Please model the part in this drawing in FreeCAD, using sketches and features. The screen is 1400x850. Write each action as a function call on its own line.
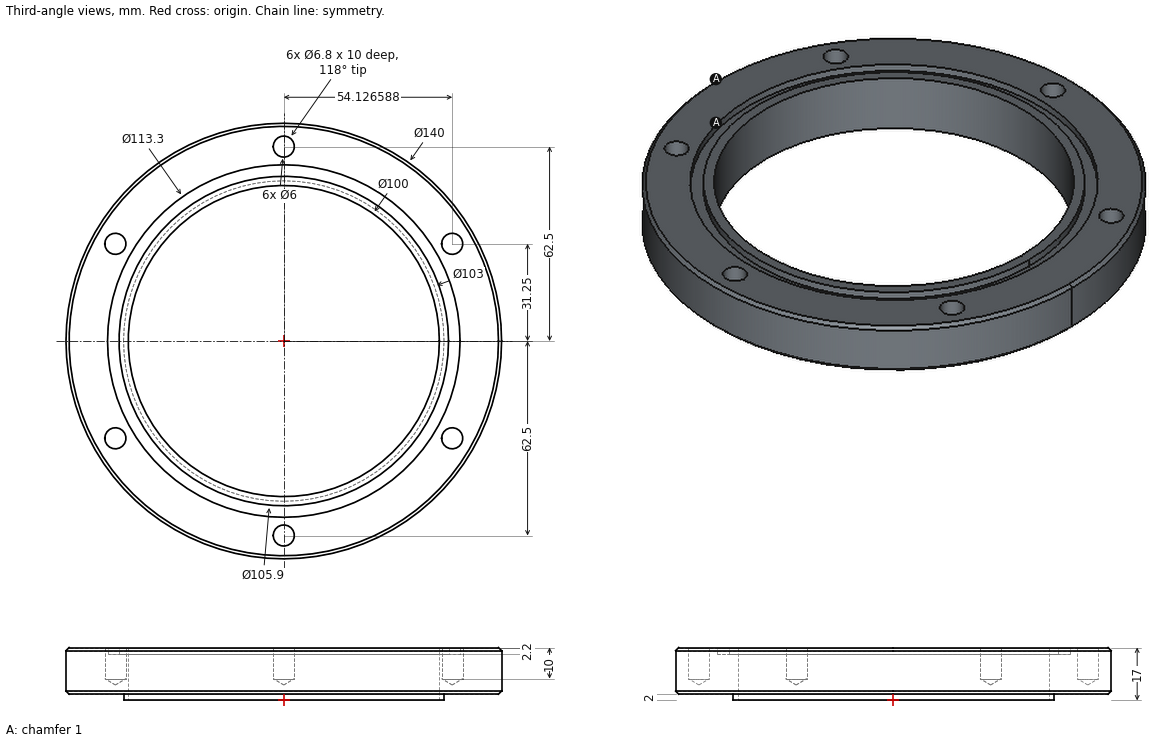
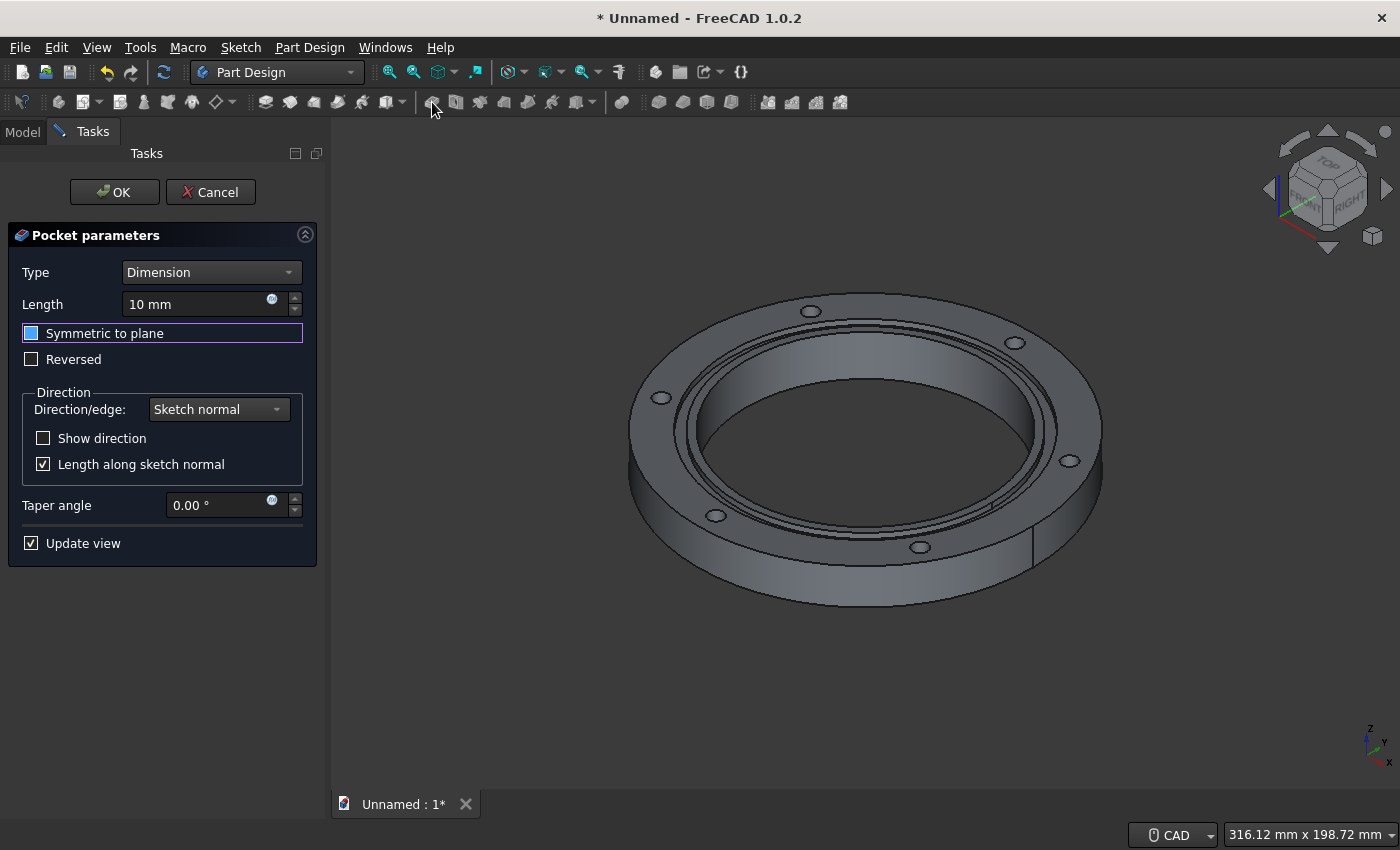
click(115, 192)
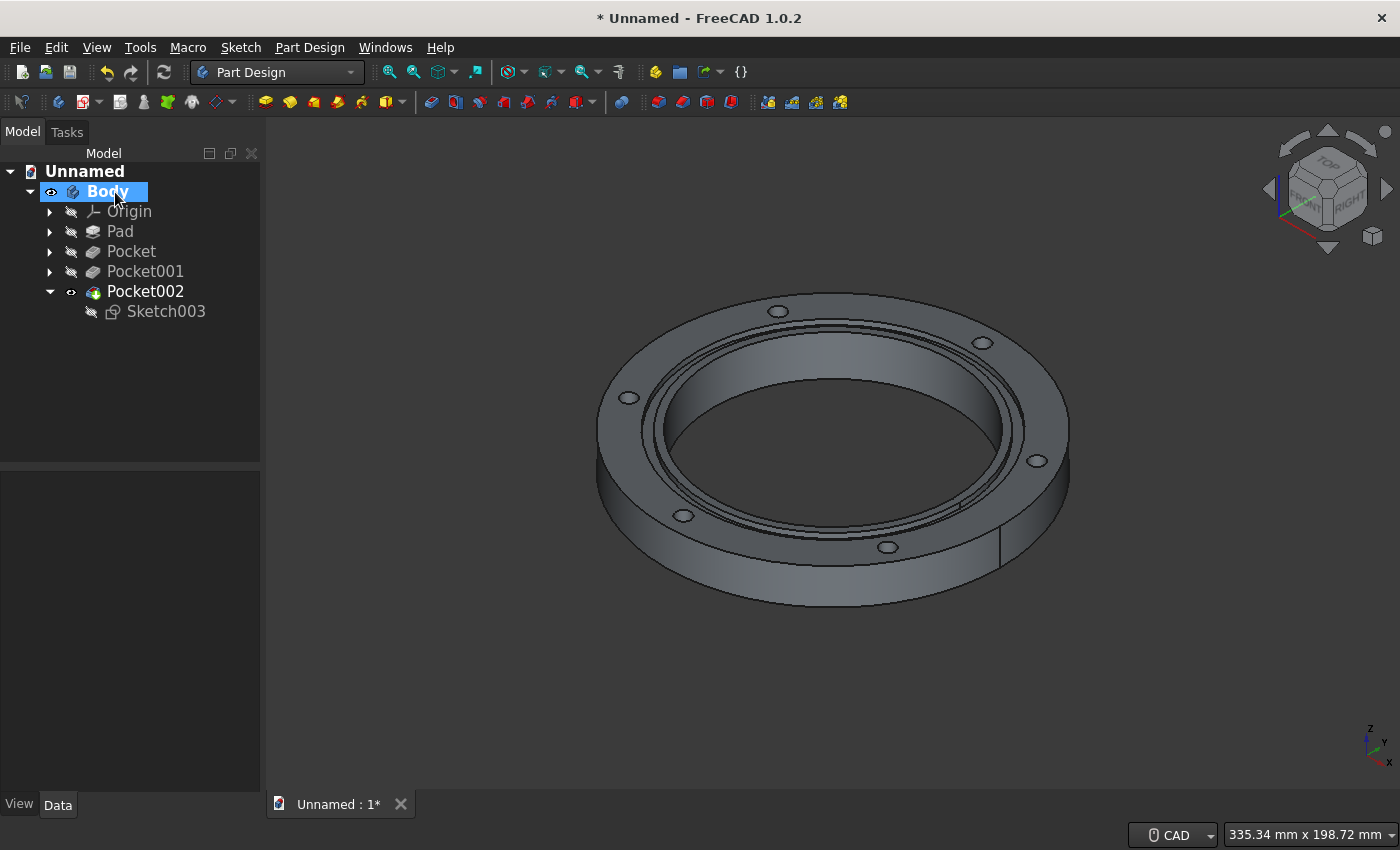
click(1024, 373)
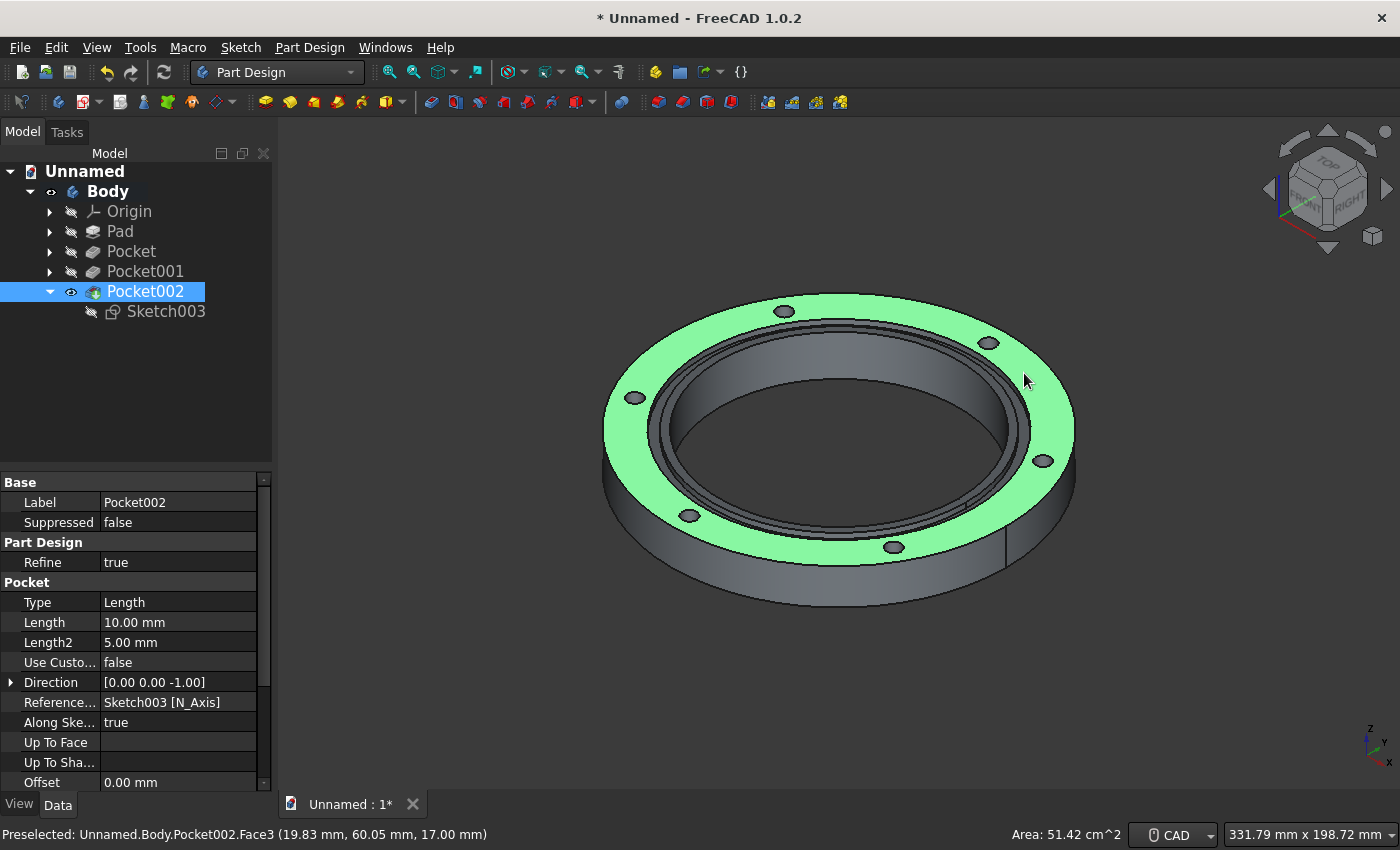
click(84, 102)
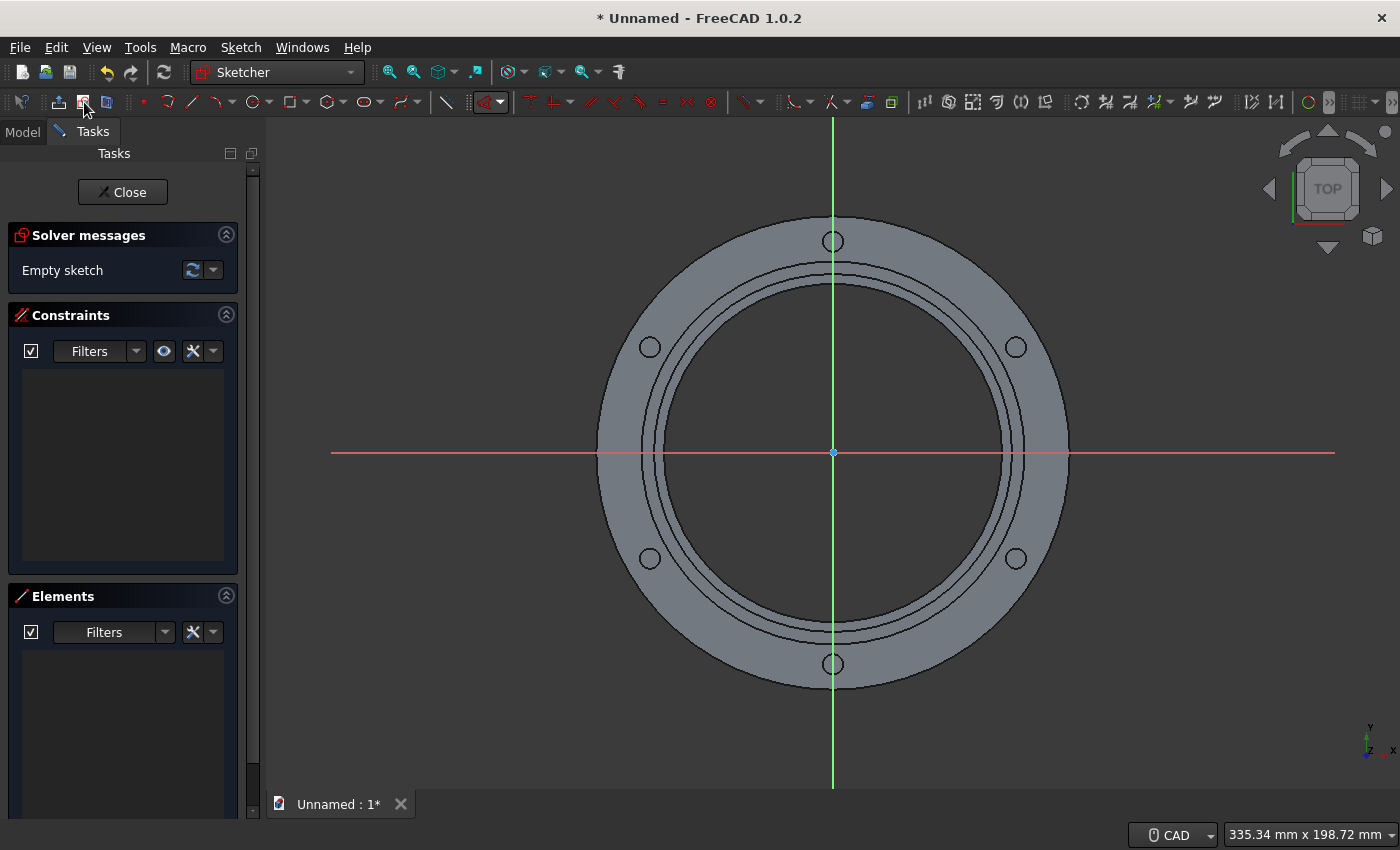
click(254, 102)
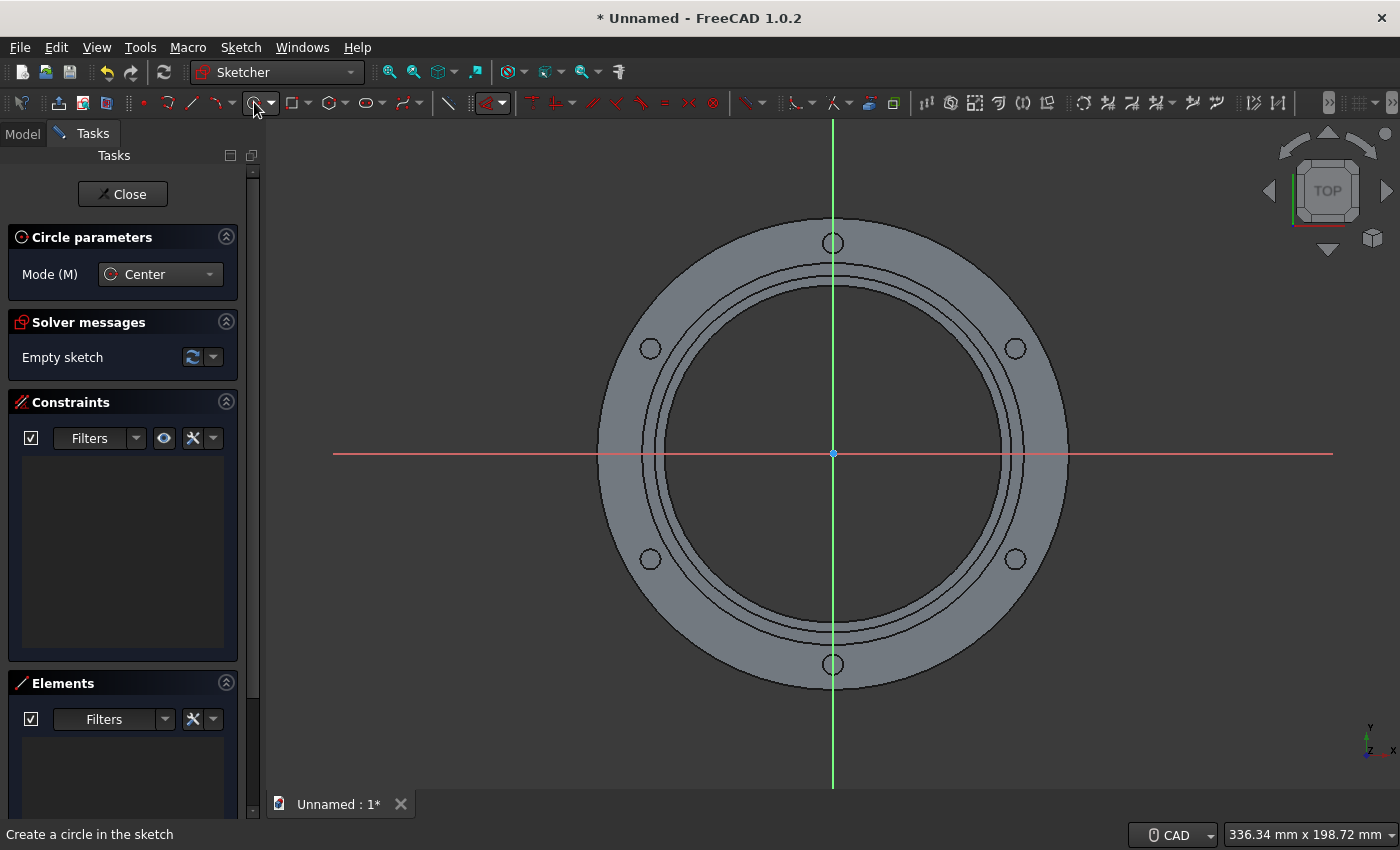
scroll(833, 243, up, 4)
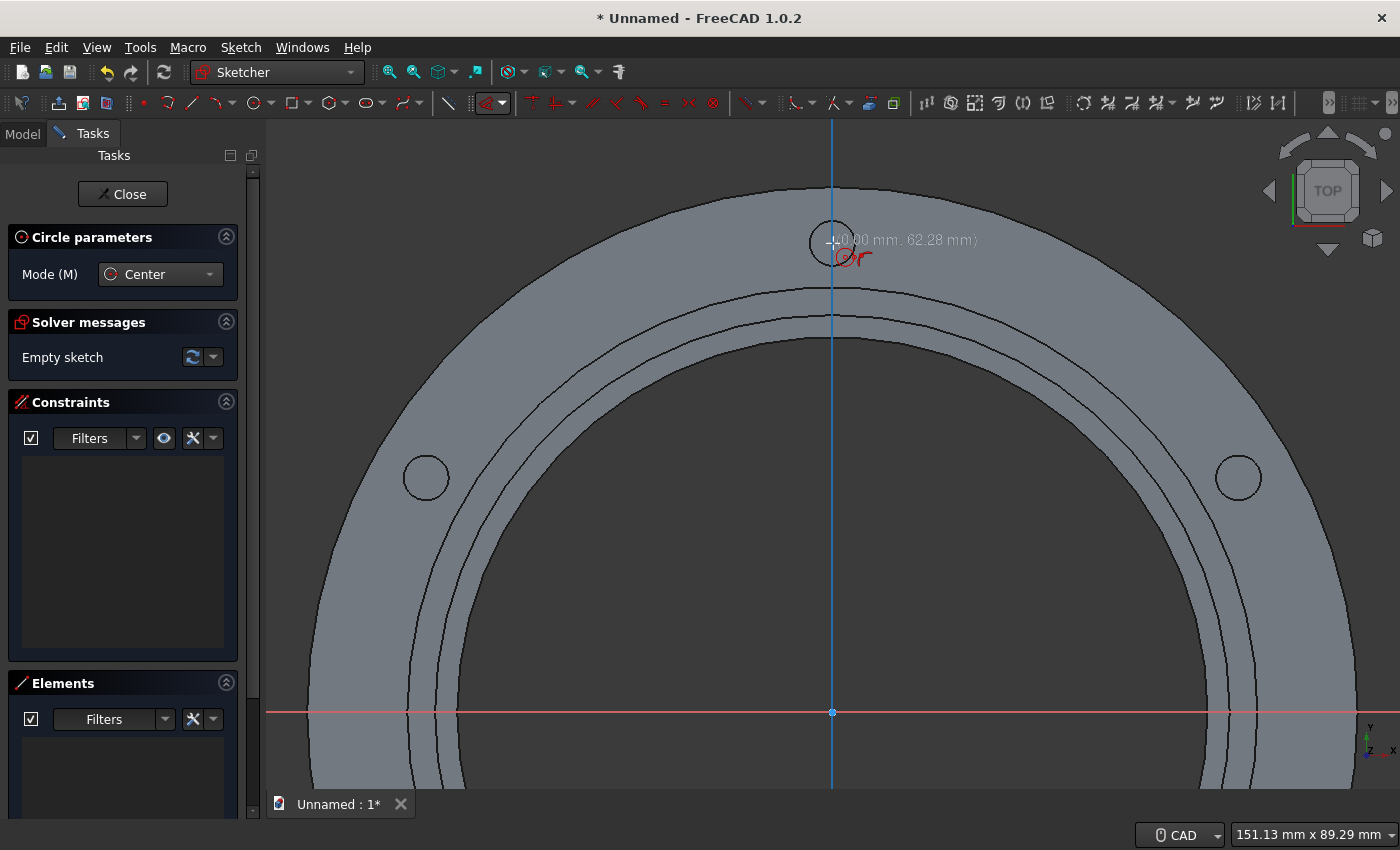
click(832, 243)
move(850, 225)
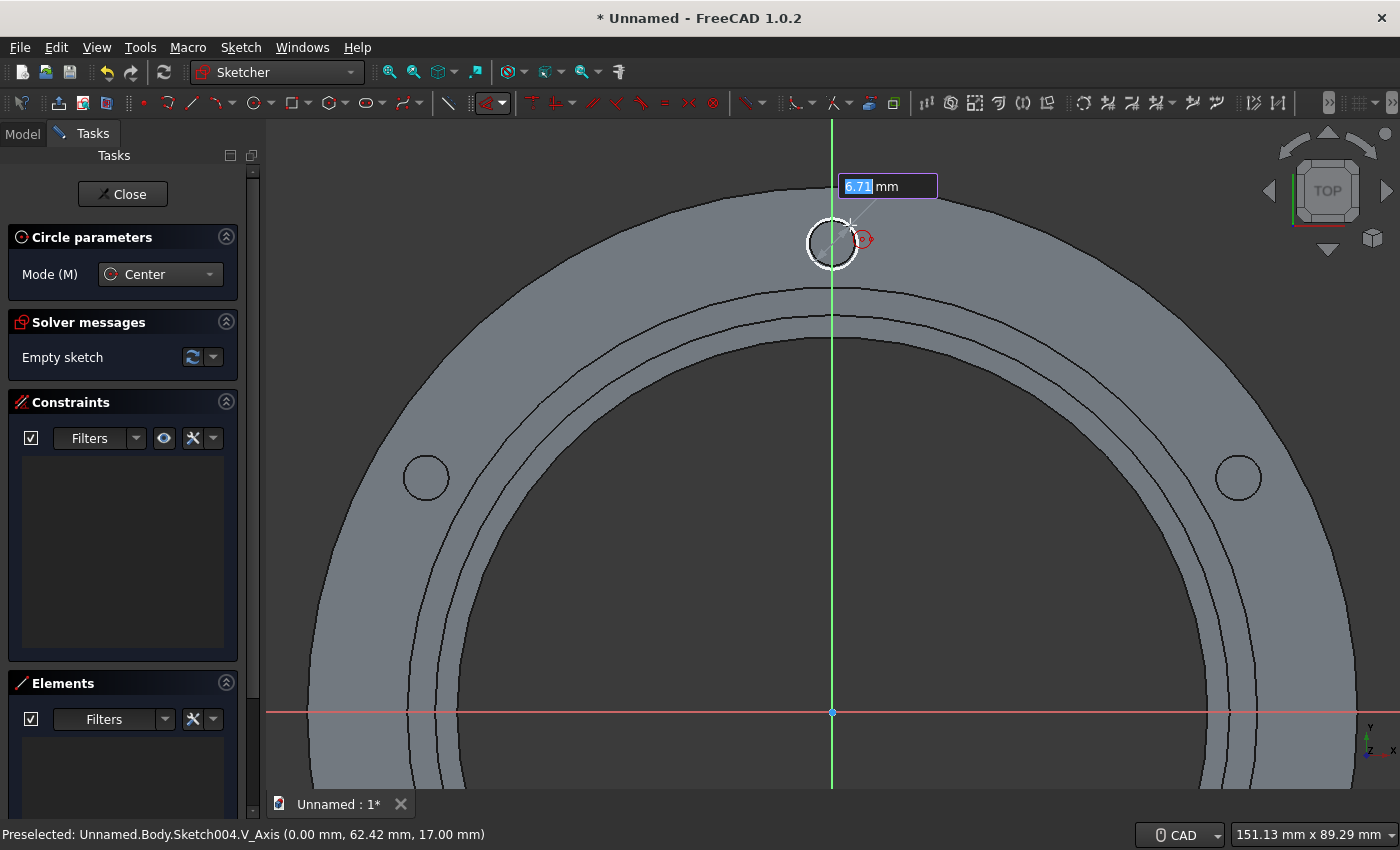
text(6.8)
key(Return)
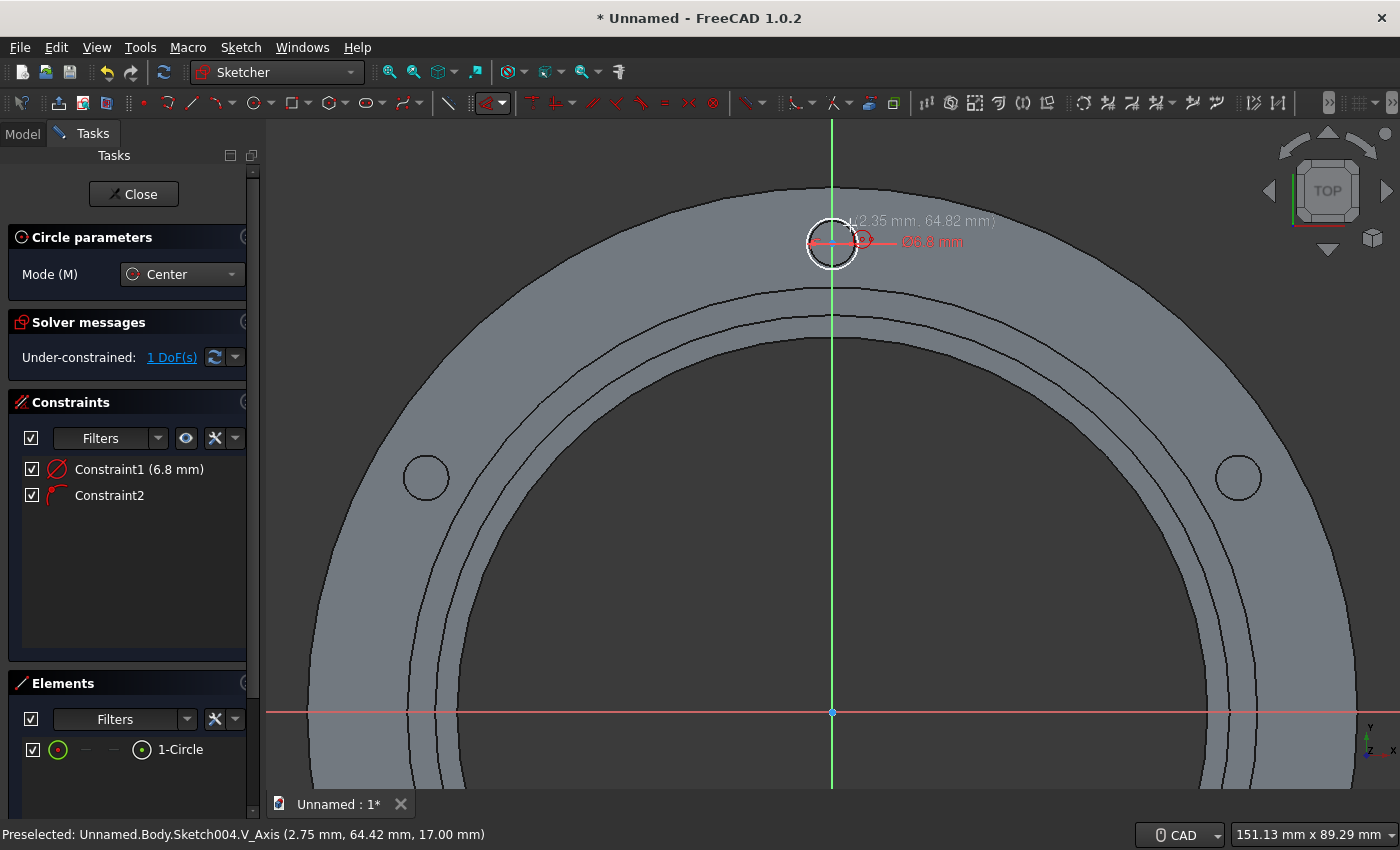
scroll(709, 243, down, 4)